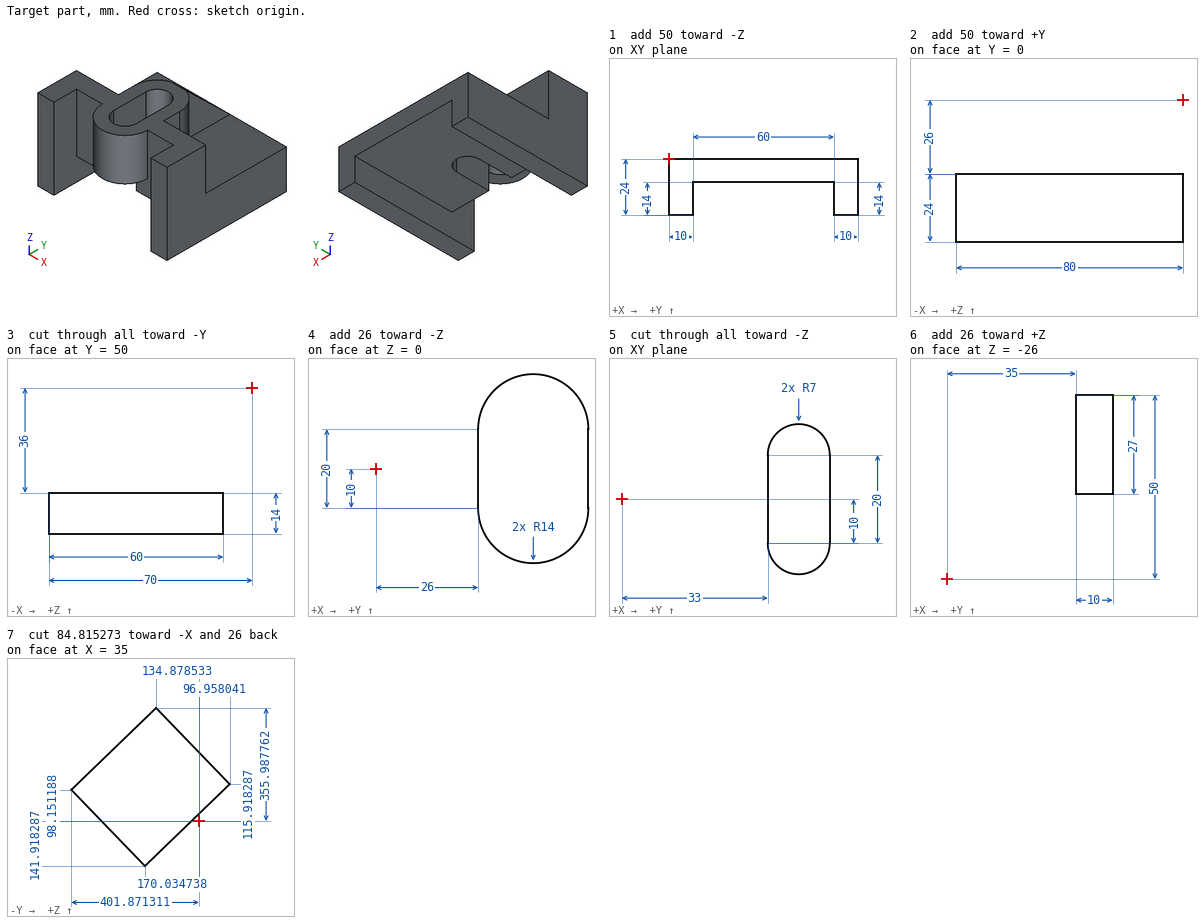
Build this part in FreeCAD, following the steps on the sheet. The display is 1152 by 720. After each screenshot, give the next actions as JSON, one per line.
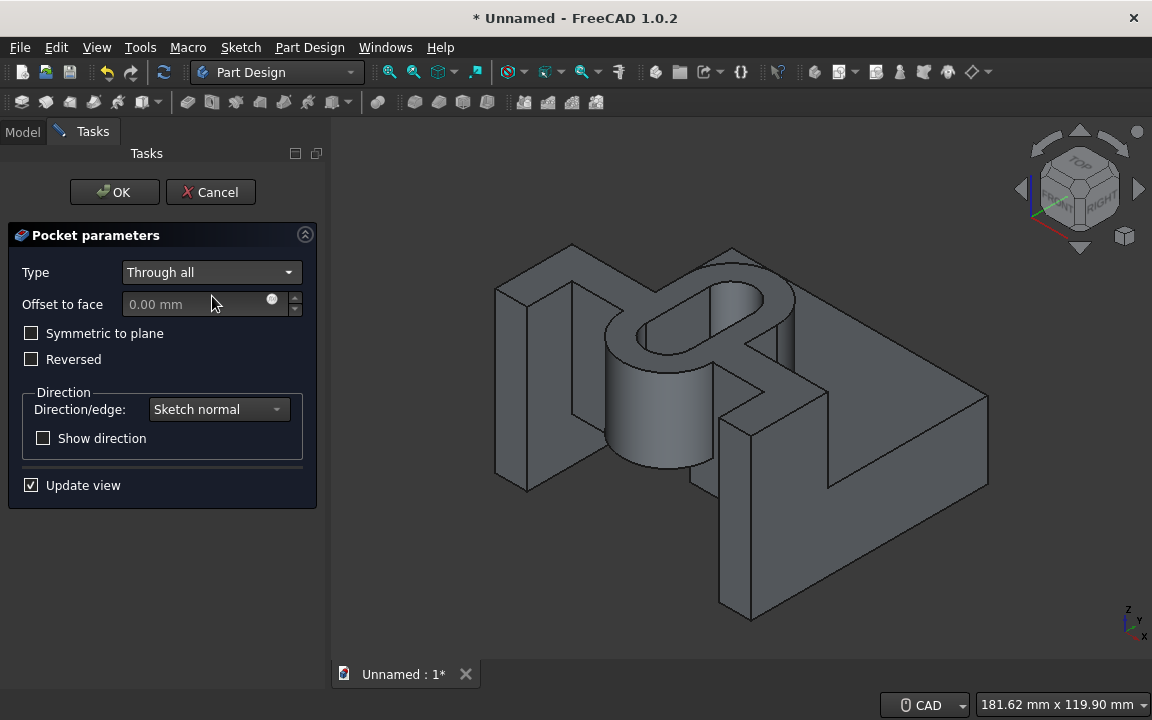
{"action": "left_click", "coordinate": [115, 192]}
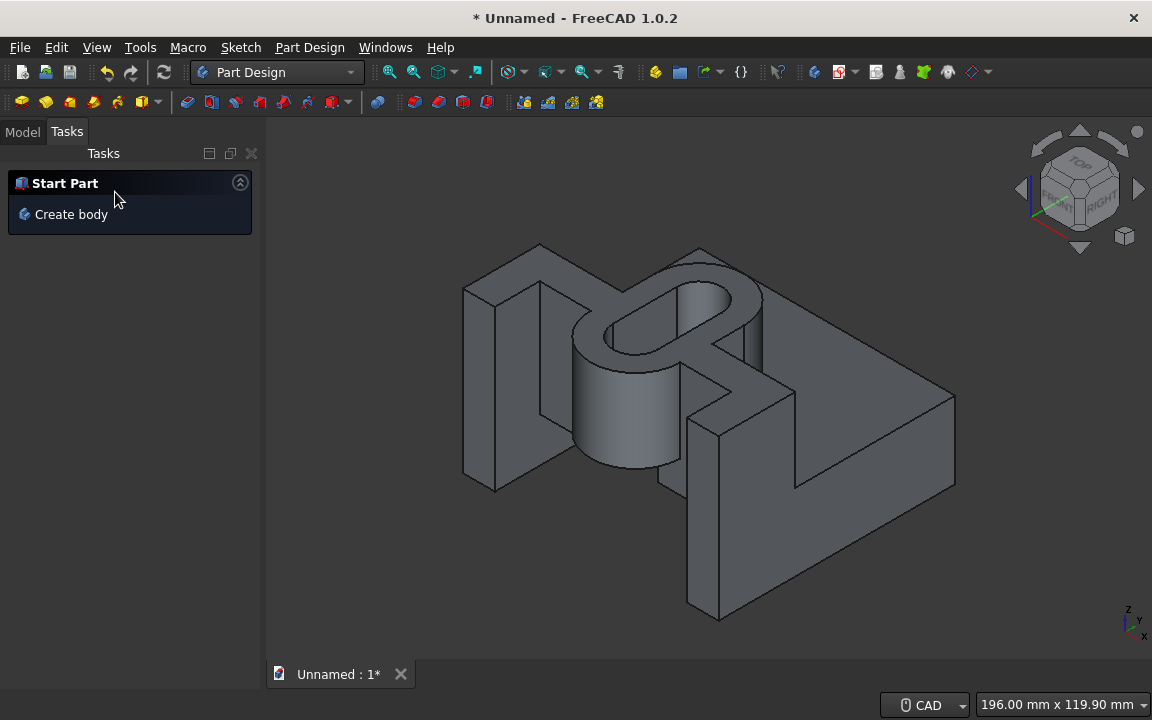
{"action": "left_click", "coordinate": [843, 396]}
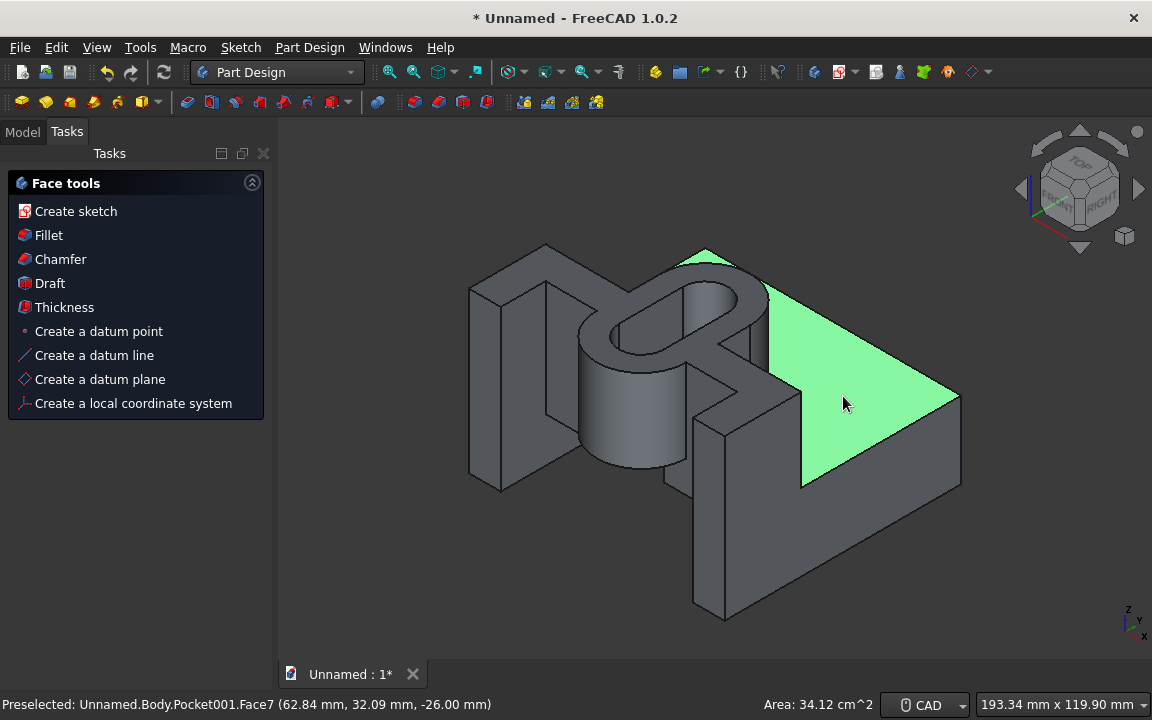
{"action": "left_click", "coordinate": [840, 72]}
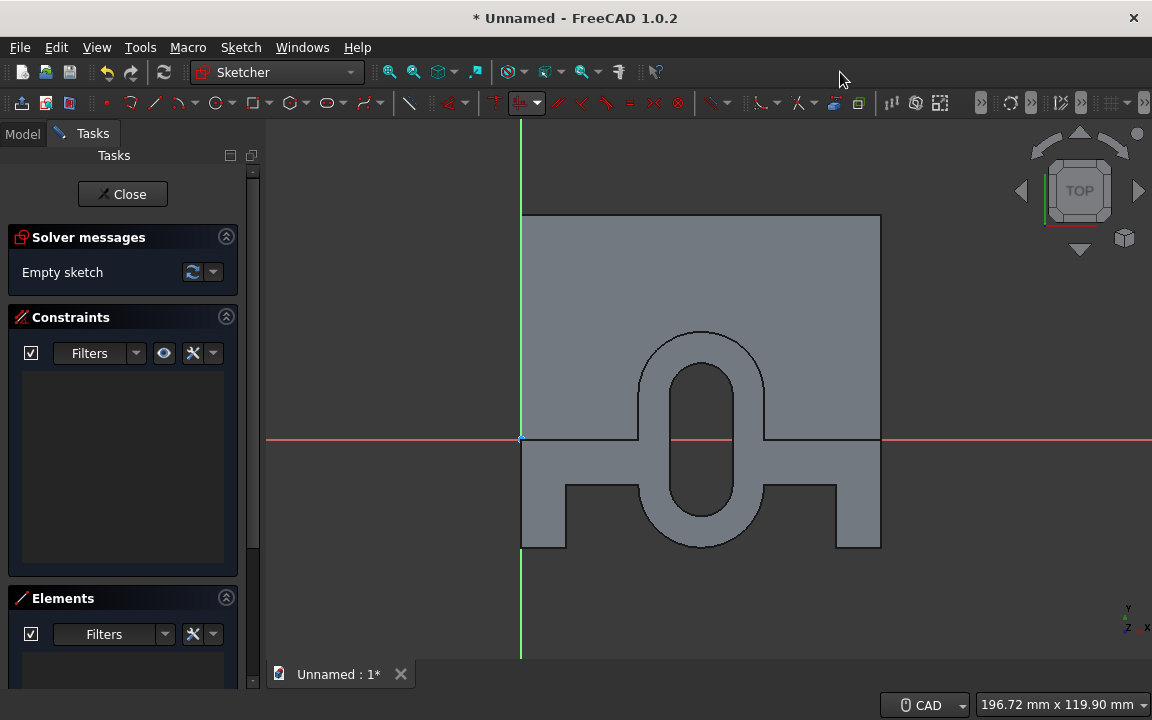
{"action": "scroll", "coordinate": [586, 202], "scroll_direction": "up", "scroll_amount": 2}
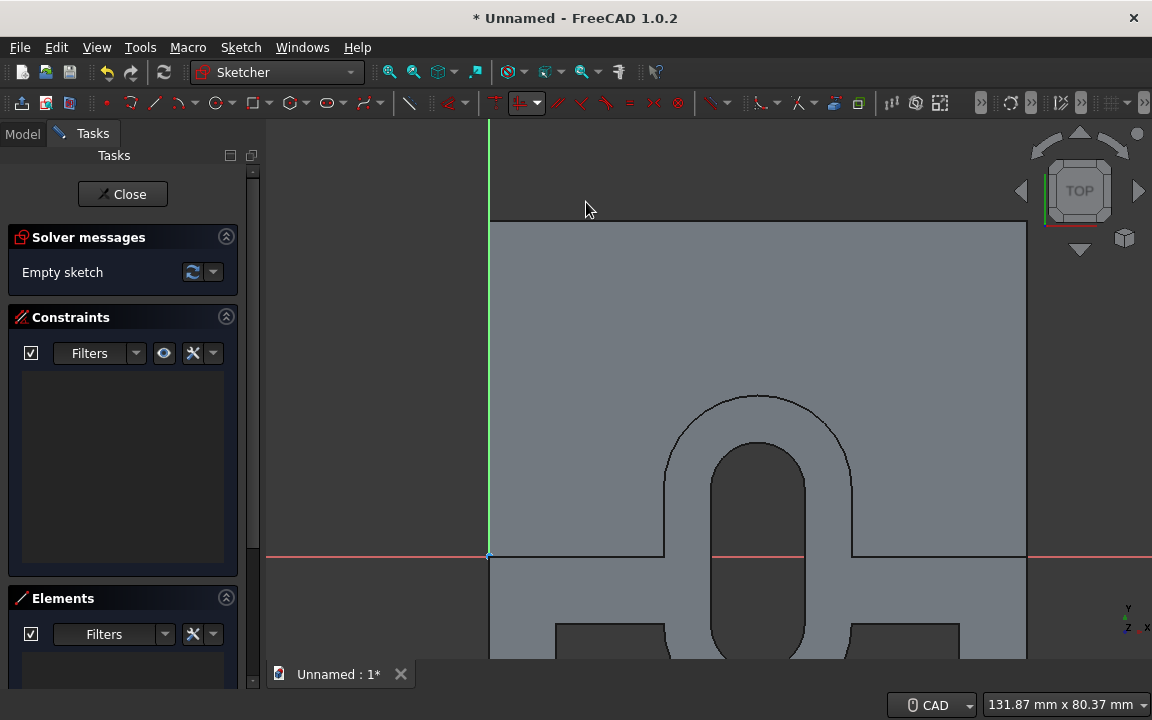
{"action": "left_click", "coordinate": [254, 104]}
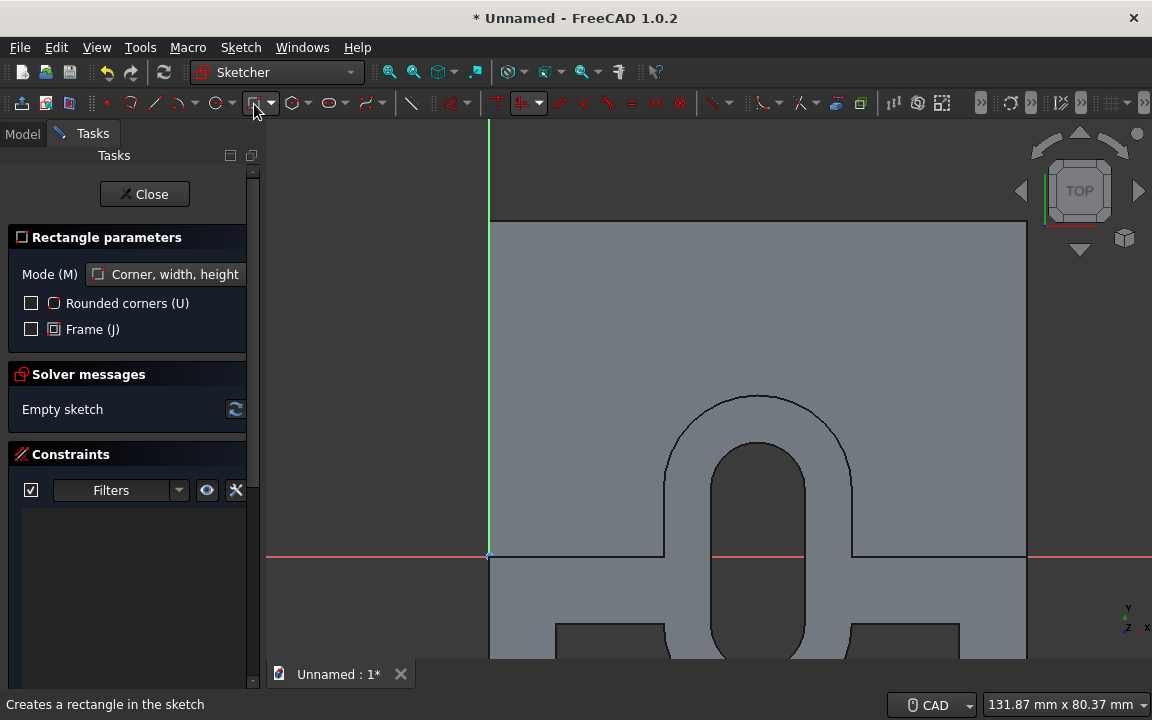
{"action": "left_click", "coordinate": [724, 221]}
{"action": "mouse_move", "coordinate": [791, 402]}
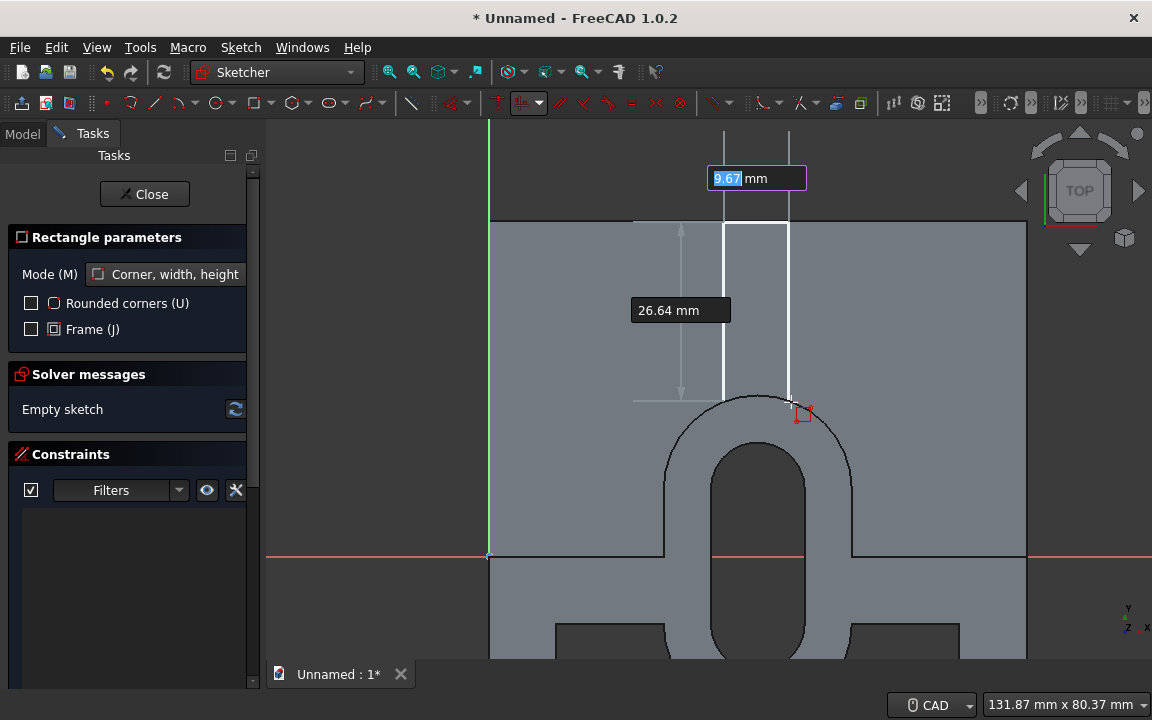
{"action": "type", "text": "10"}
{"action": "key", "text": "Tab"}
{"action": "type", "text": "27"}
{"action": "key", "text": "Return"}
{"action": "key", "text": "Escape"}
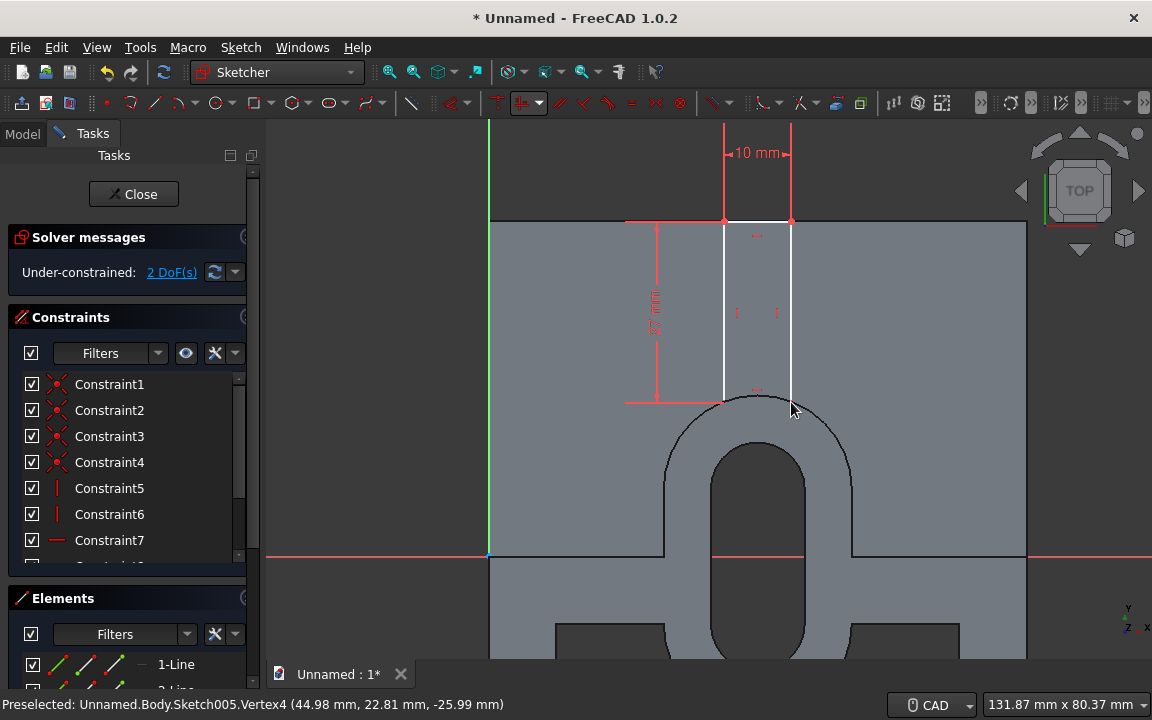
{"action": "key", "text": "d"}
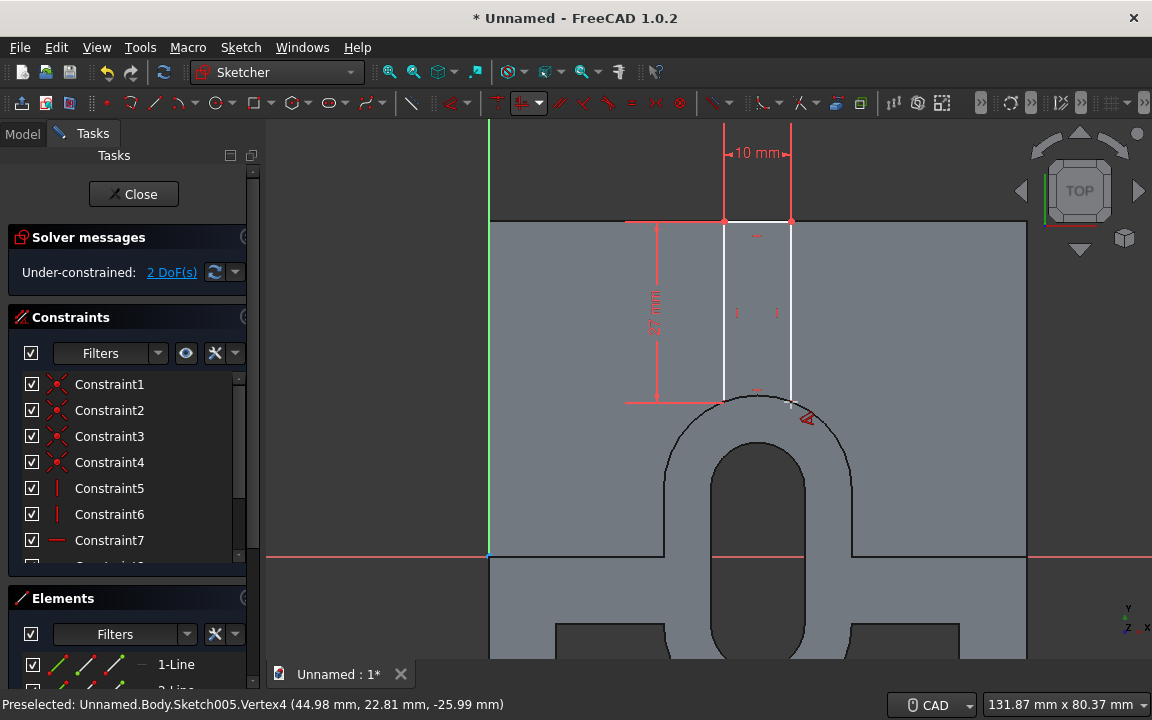
{"action": "left_click", "coordinate": [724, 222]}
{"action": "left_click", "coordinate": [607, 591]}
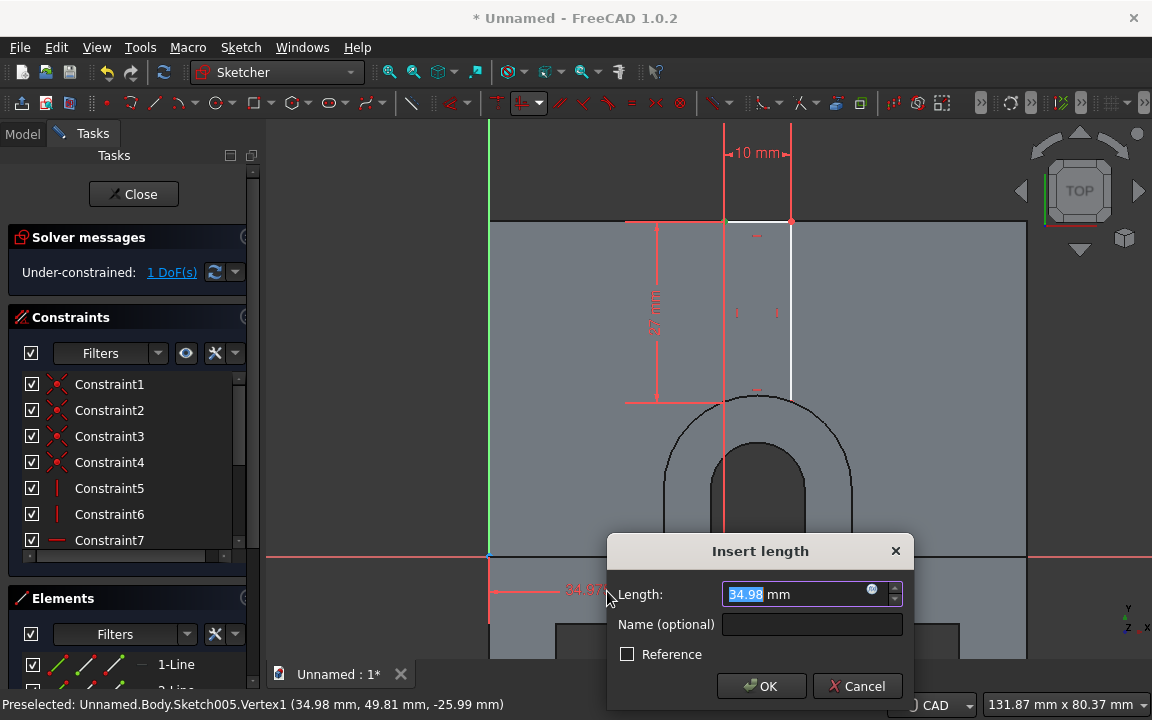
{"action": "type", "text": "35"}
{"action": "key", "text": "Return"}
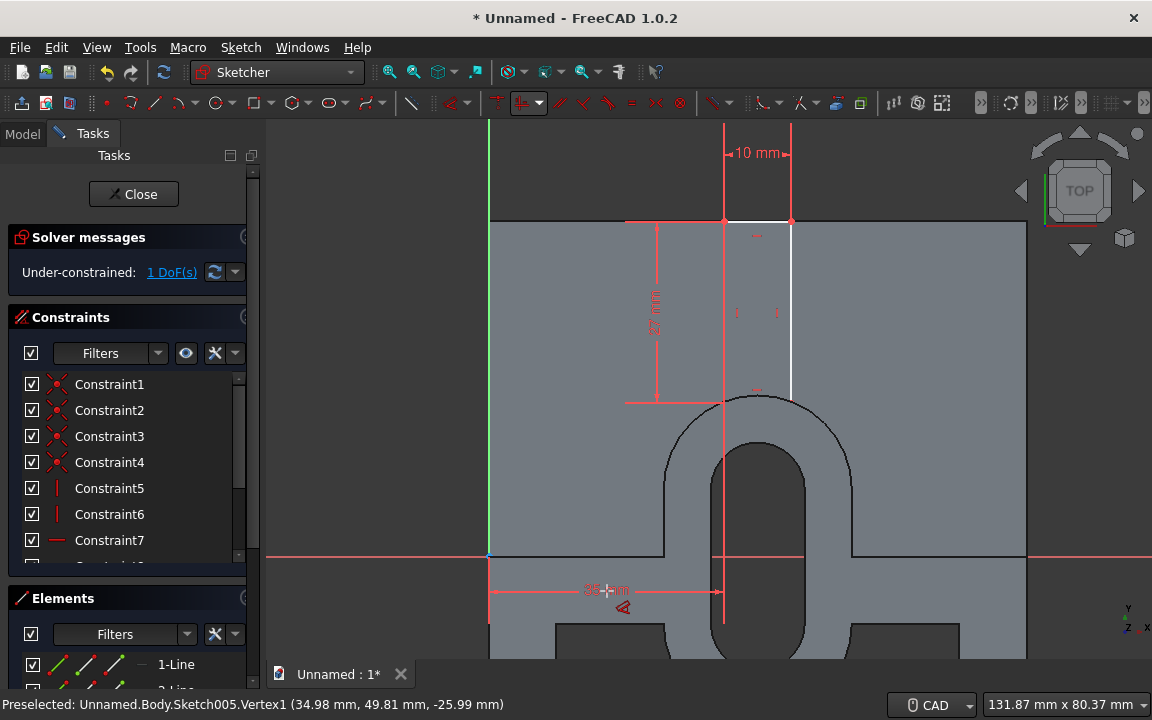
{"action": "left_click", "coordinate": [724, 222]}
{"action": "left_click", "coordinate": [455, 389]}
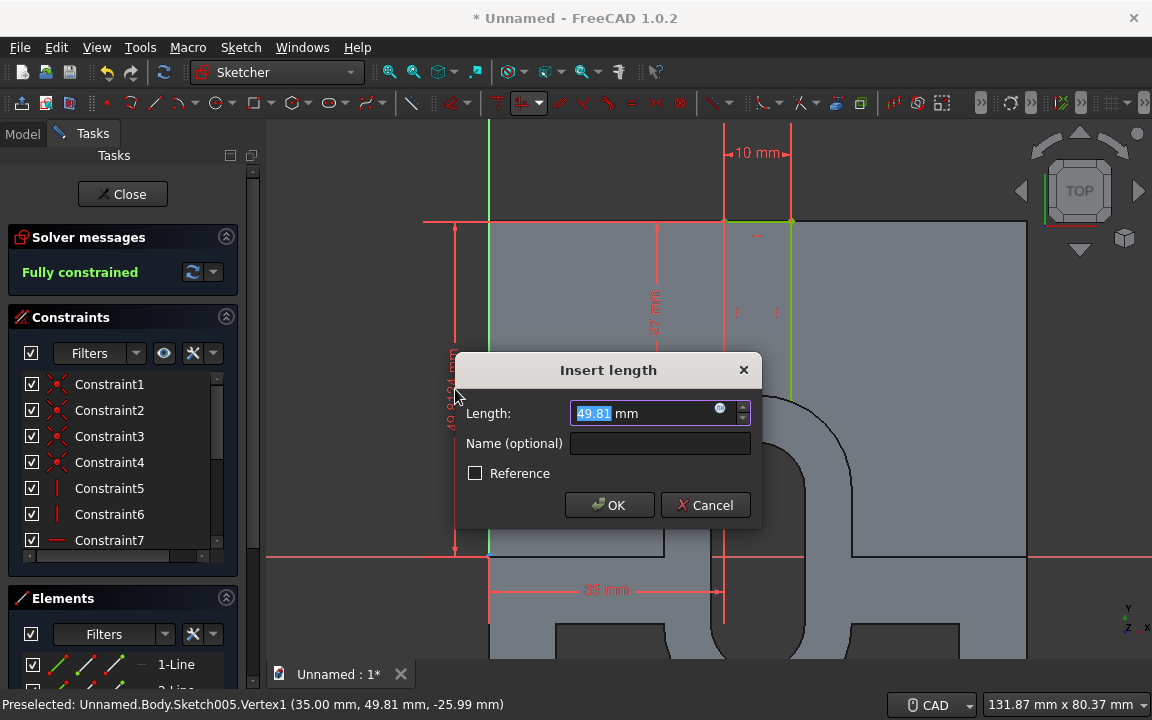
{"action": "type", "text": "50"}
{"action": "key", "text": "Return"}
{"action": "key", "text": "Escape"}